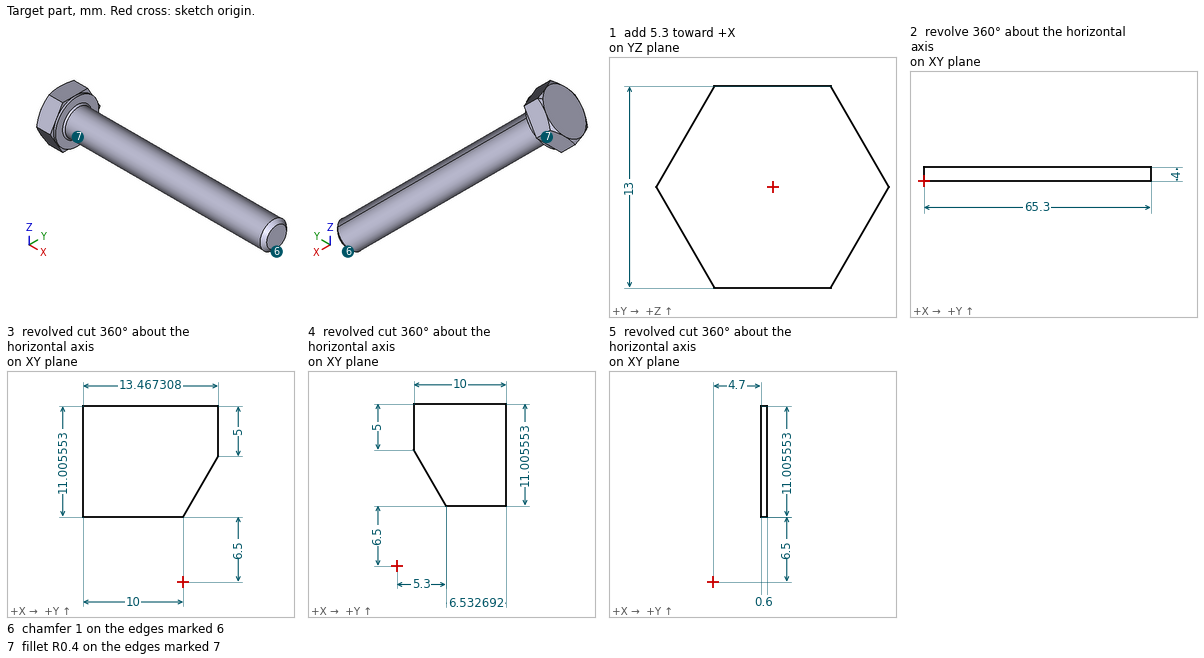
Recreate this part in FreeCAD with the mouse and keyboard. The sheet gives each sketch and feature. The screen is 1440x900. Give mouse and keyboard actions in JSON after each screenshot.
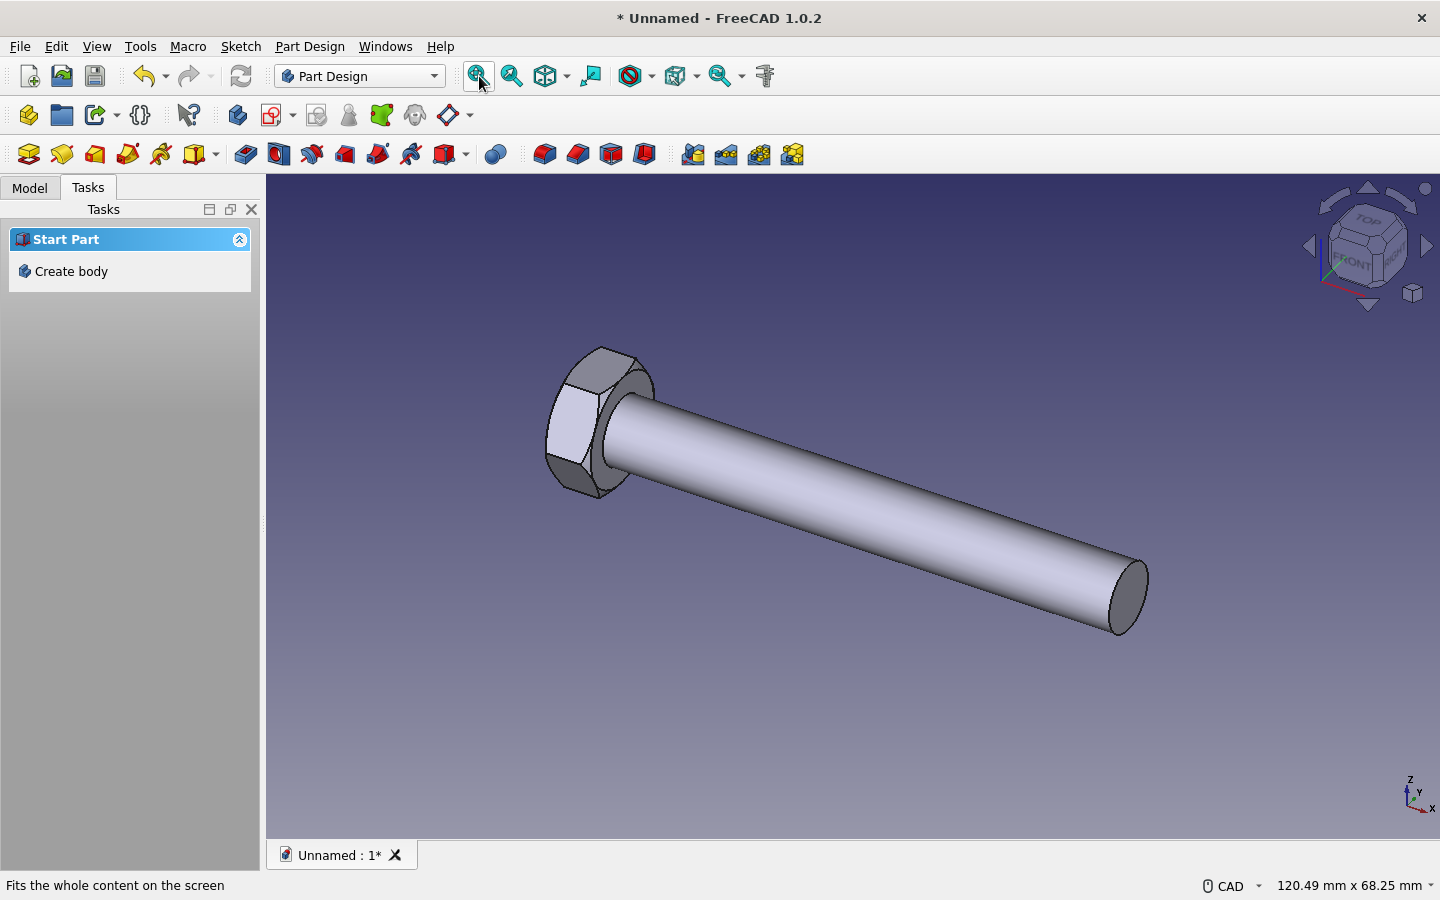
{"action": "left_click", "coordinate": [270, 116]}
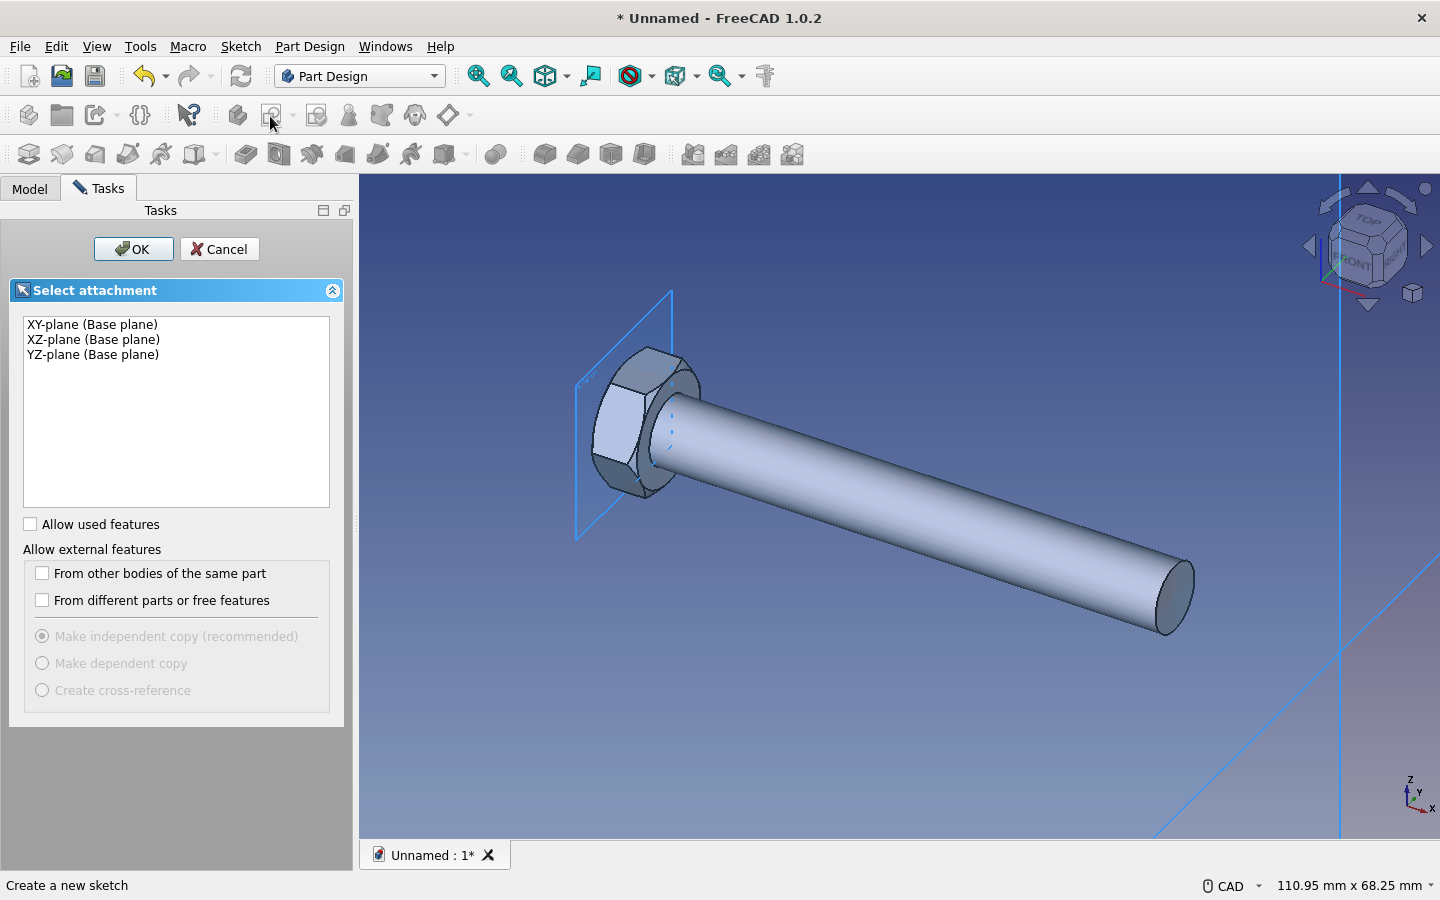
{"action": "left_click", "coordinate": [84, 324]}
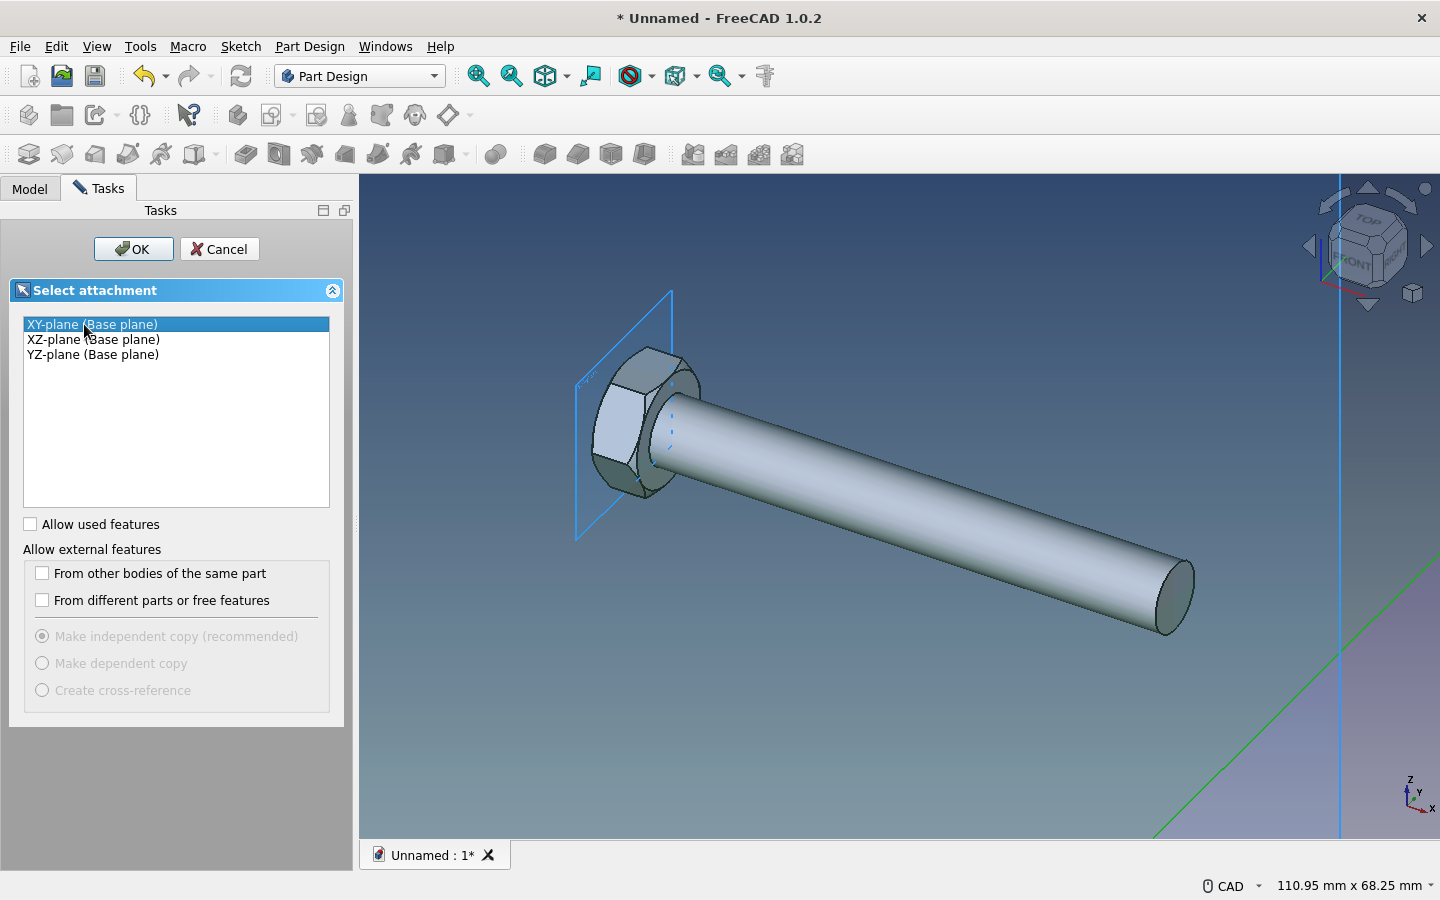
{"action": "left_click", "coordinate": [134, 249]}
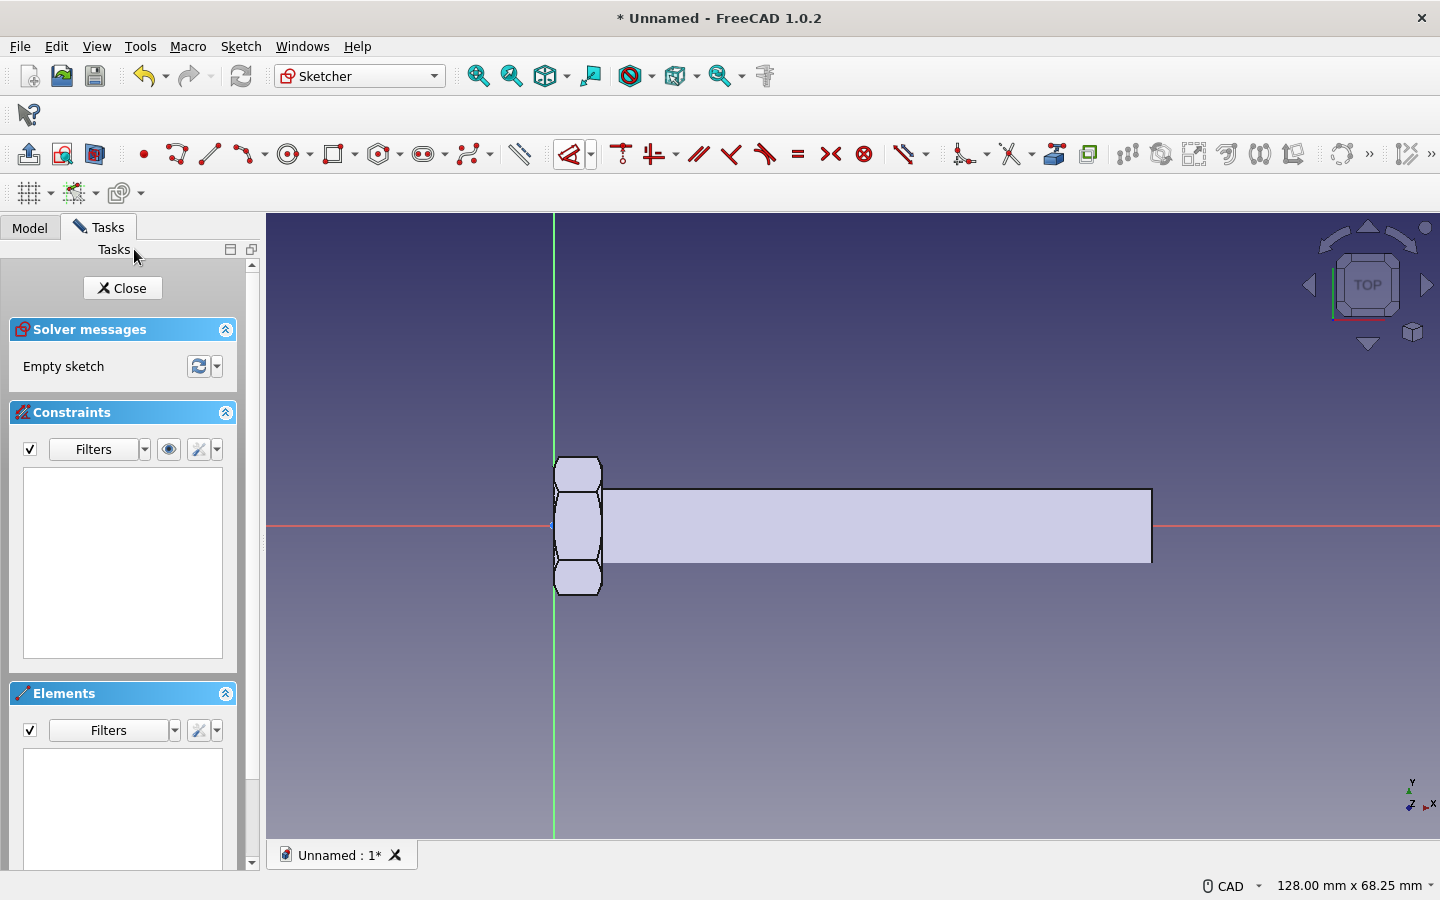
{"action": "left_click", "coordinate": [95, 154]}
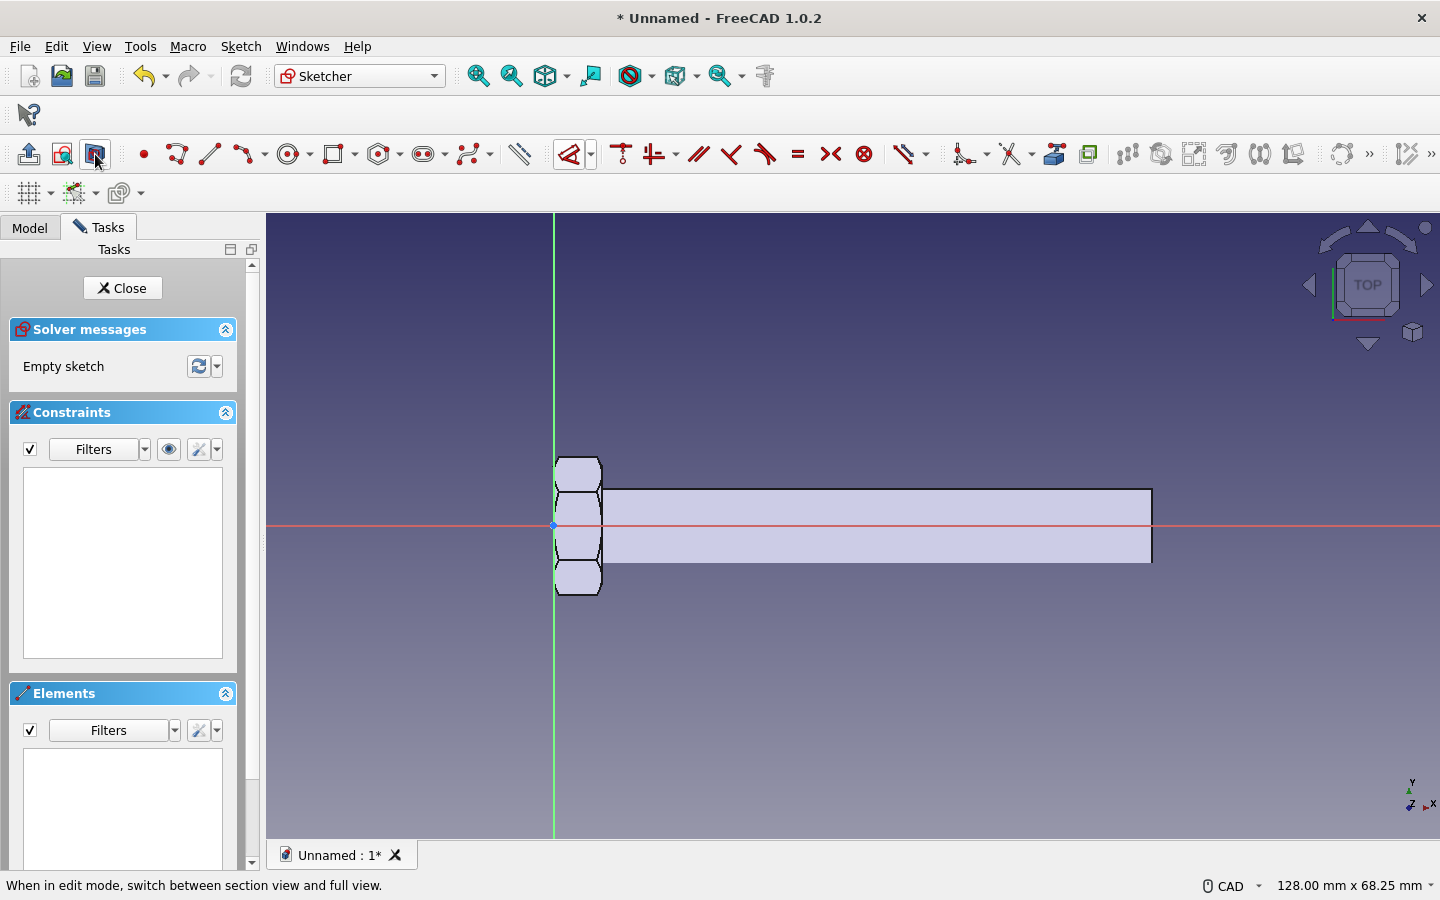
{"action": "scroll", "coordinate": [458, 399], "scroll_direction": "up", "scroll_amount": 5}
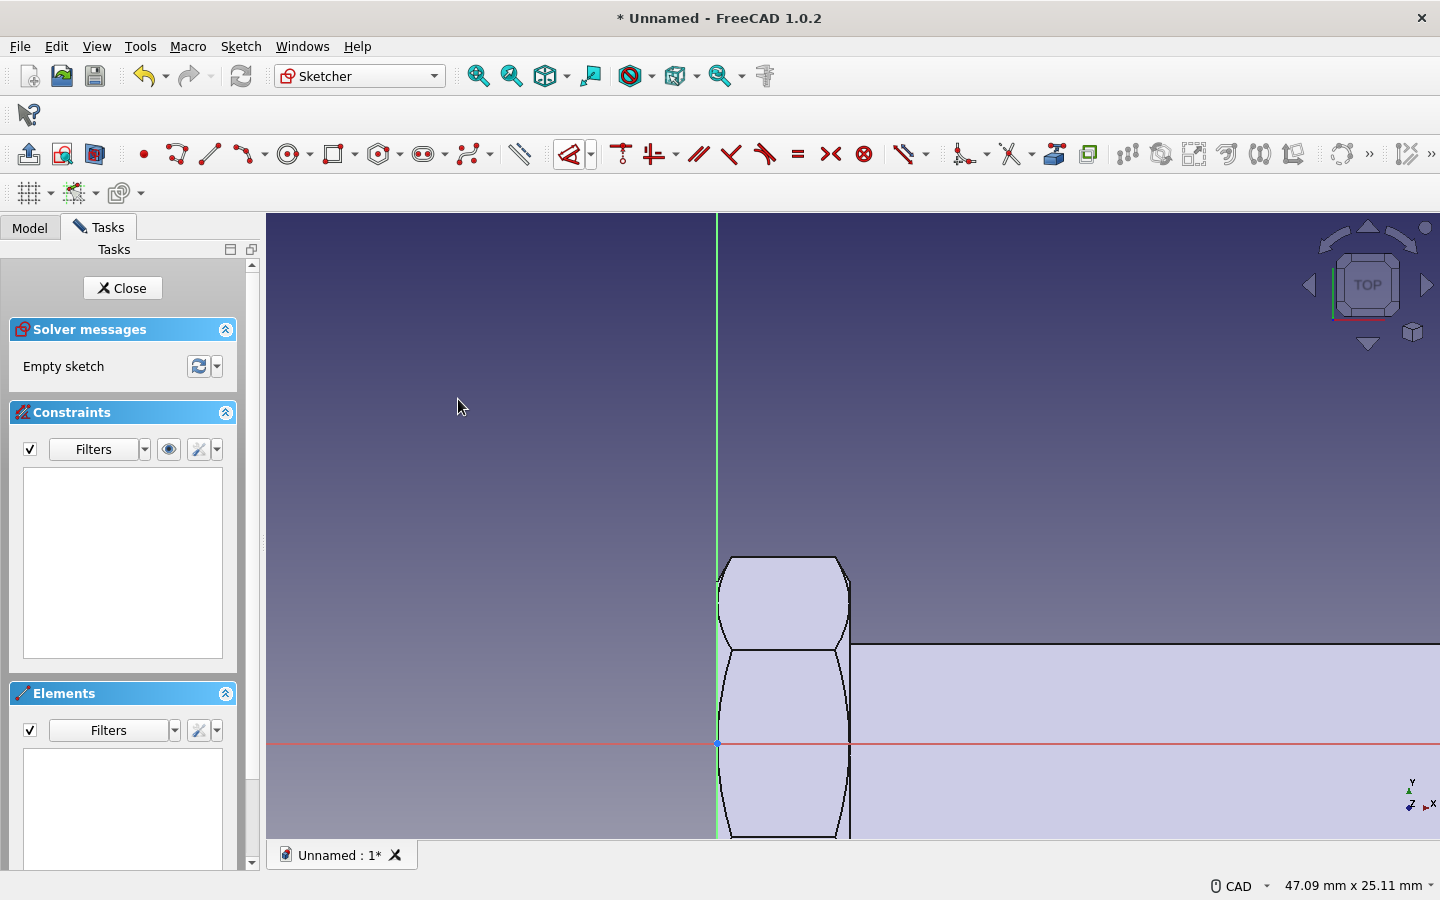
{"action": "left_click", "coordinate": [332, 154]}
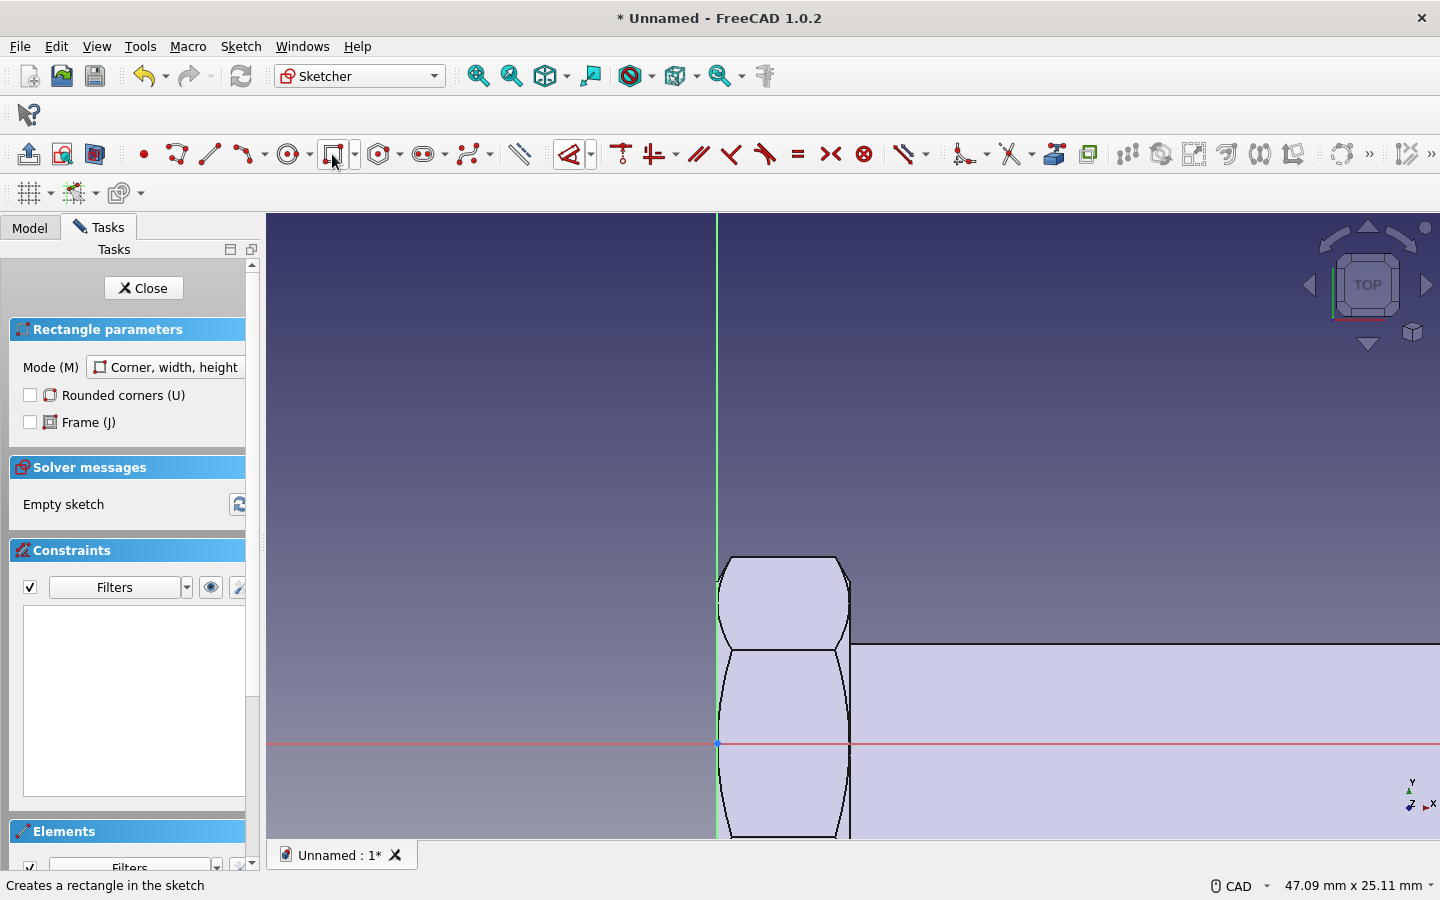
{"action": "left_click", "coordinate": [835, 307]}
{"action": "left_click", "coordinate": [850, 582]}
{"action": "key", "text": "Escape"}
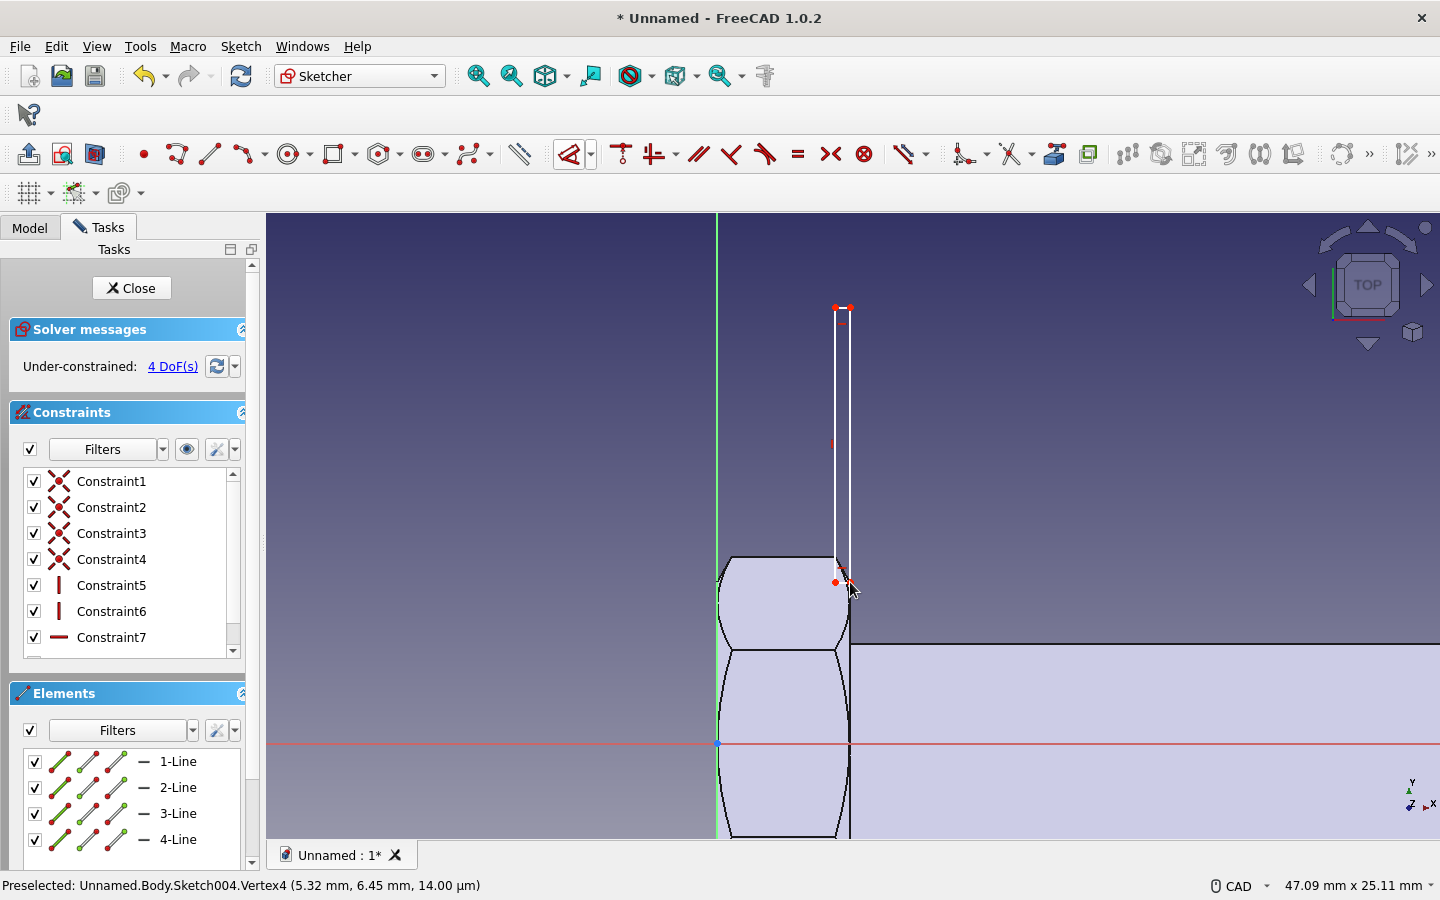
{"action": "scroll", "coordinate": [843, 583], "scroll_direction": "up", "scroll_amount": 5}